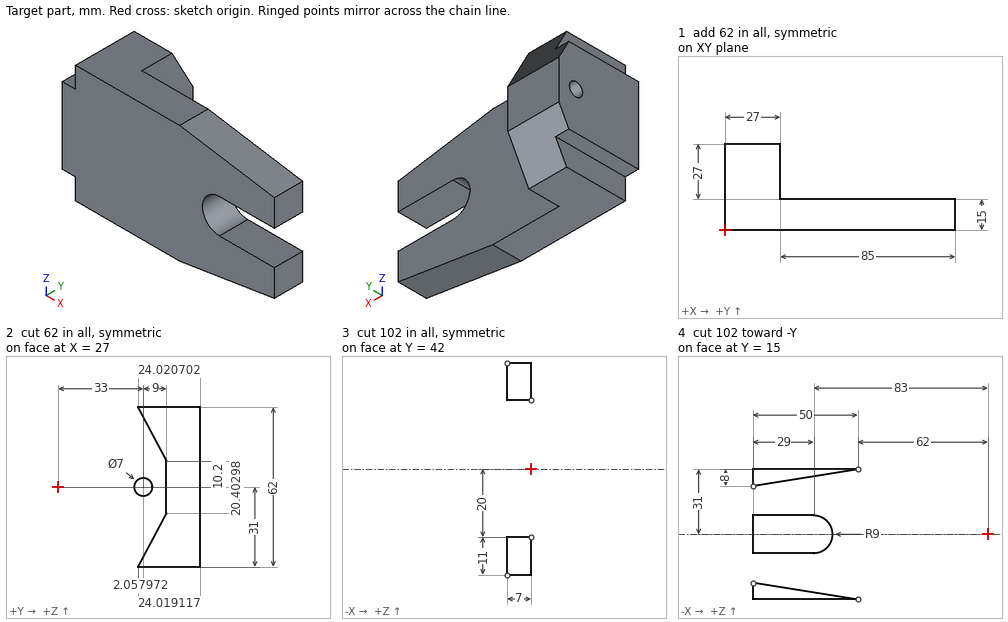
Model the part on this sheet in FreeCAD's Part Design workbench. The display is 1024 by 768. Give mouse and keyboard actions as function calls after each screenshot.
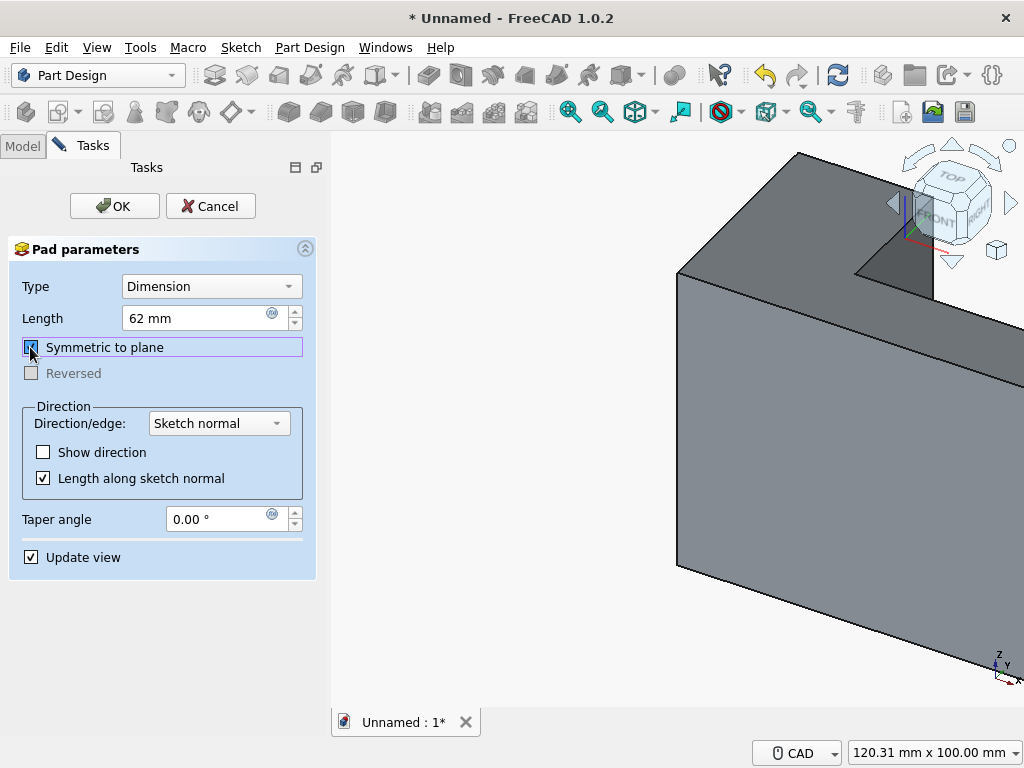
click(115, 206)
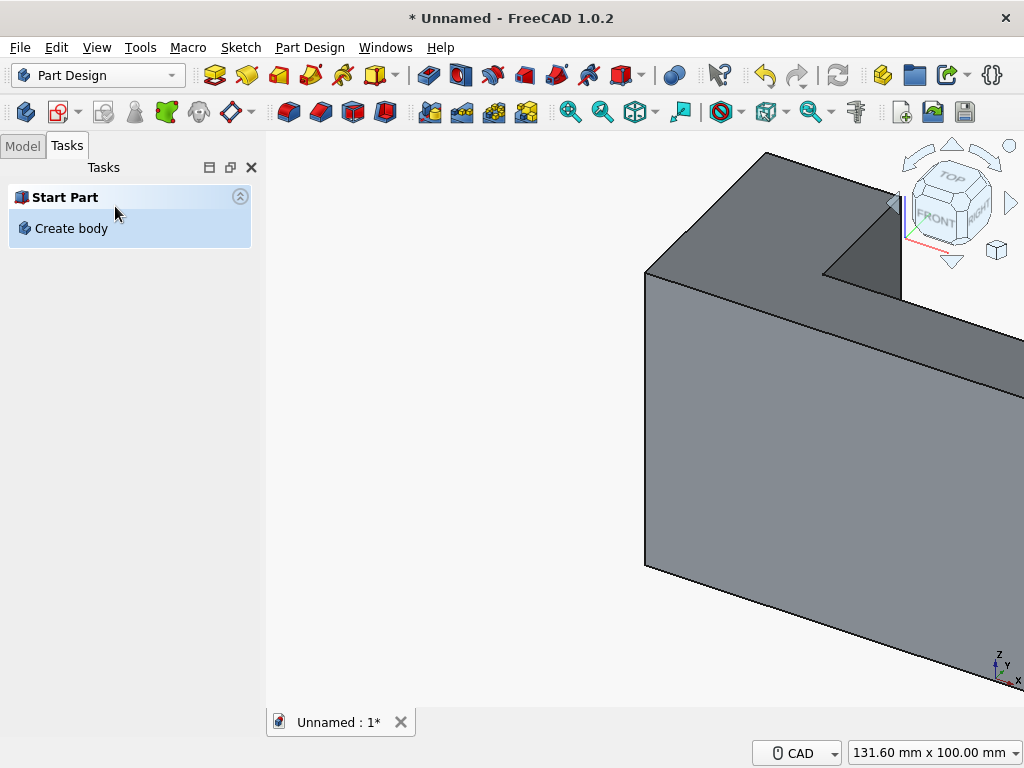
click(572, 112)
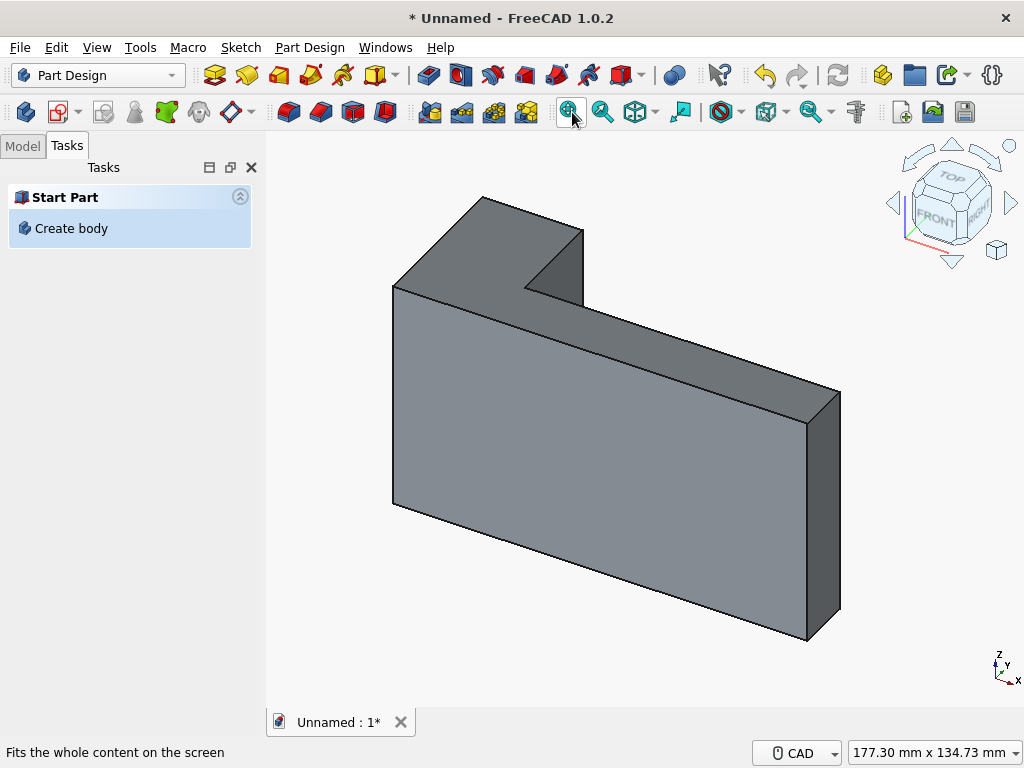
key(0)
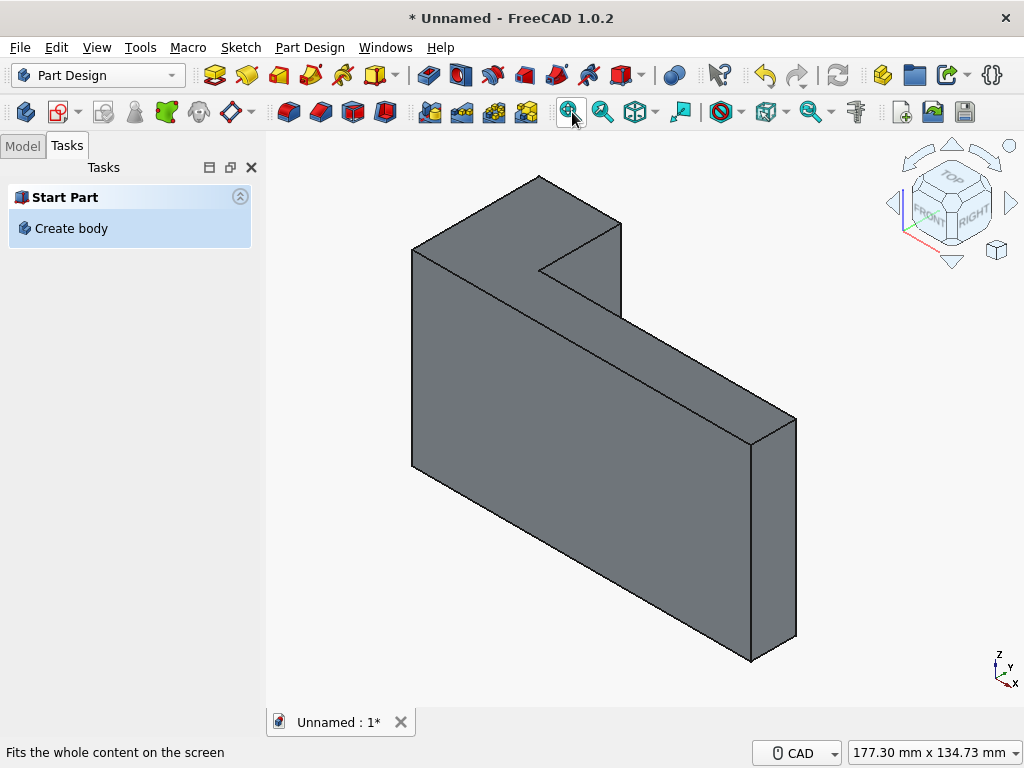
key(3)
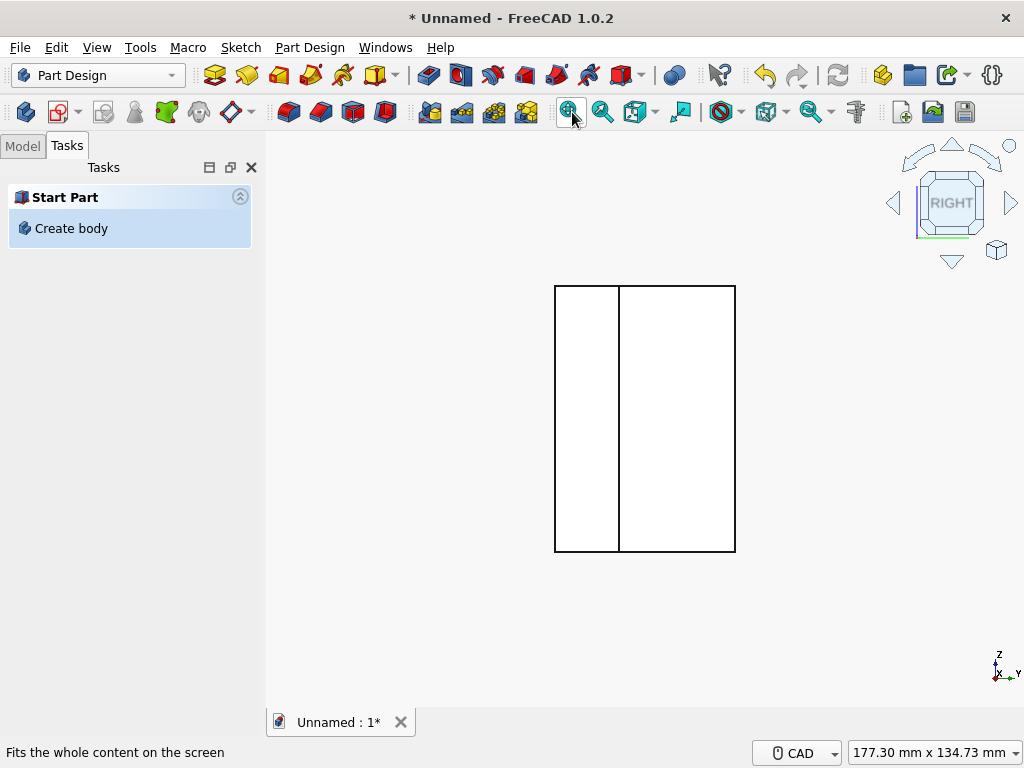
click(677, 380)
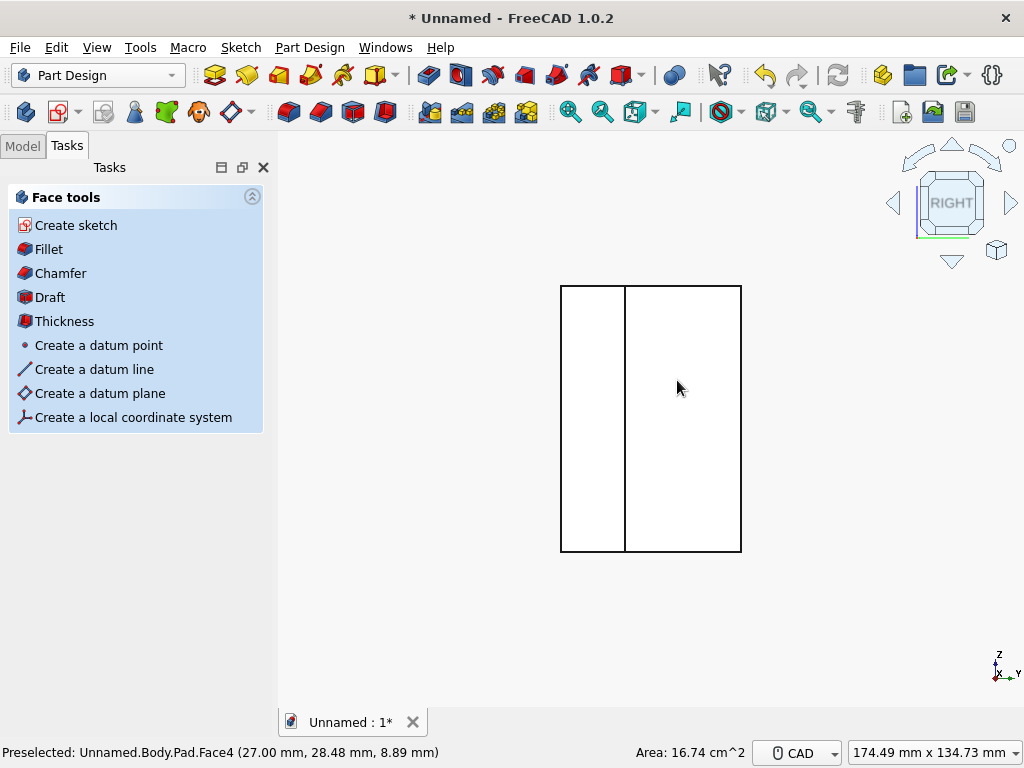
click(58, 112)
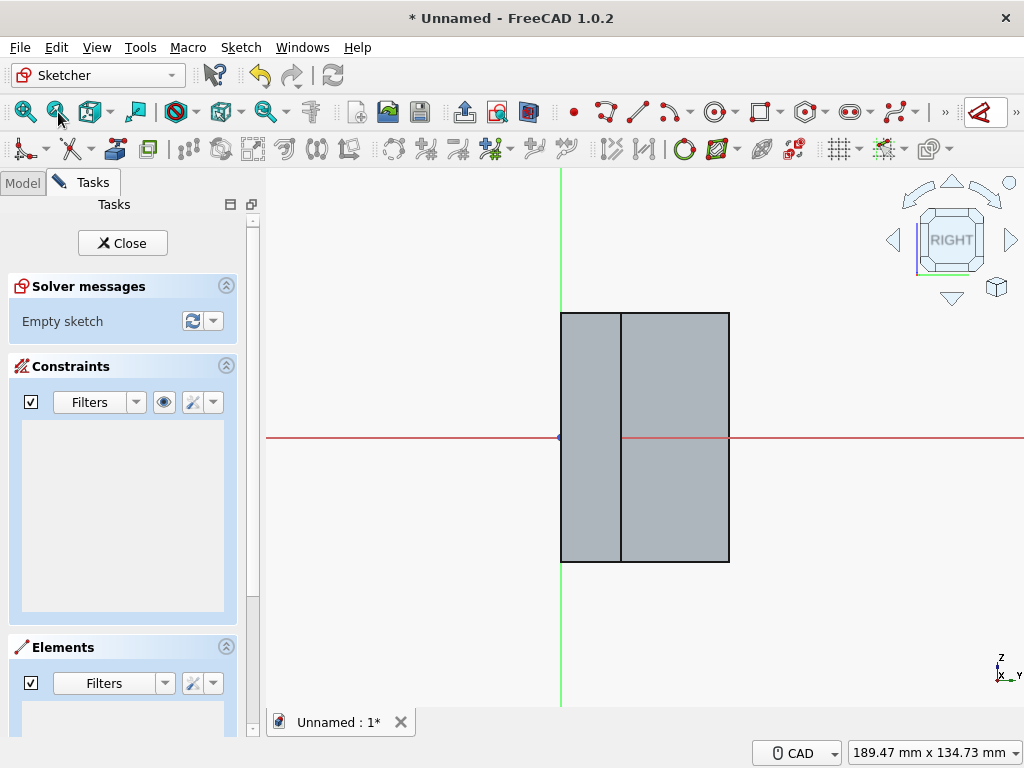
scroll(859, 438, up, 2)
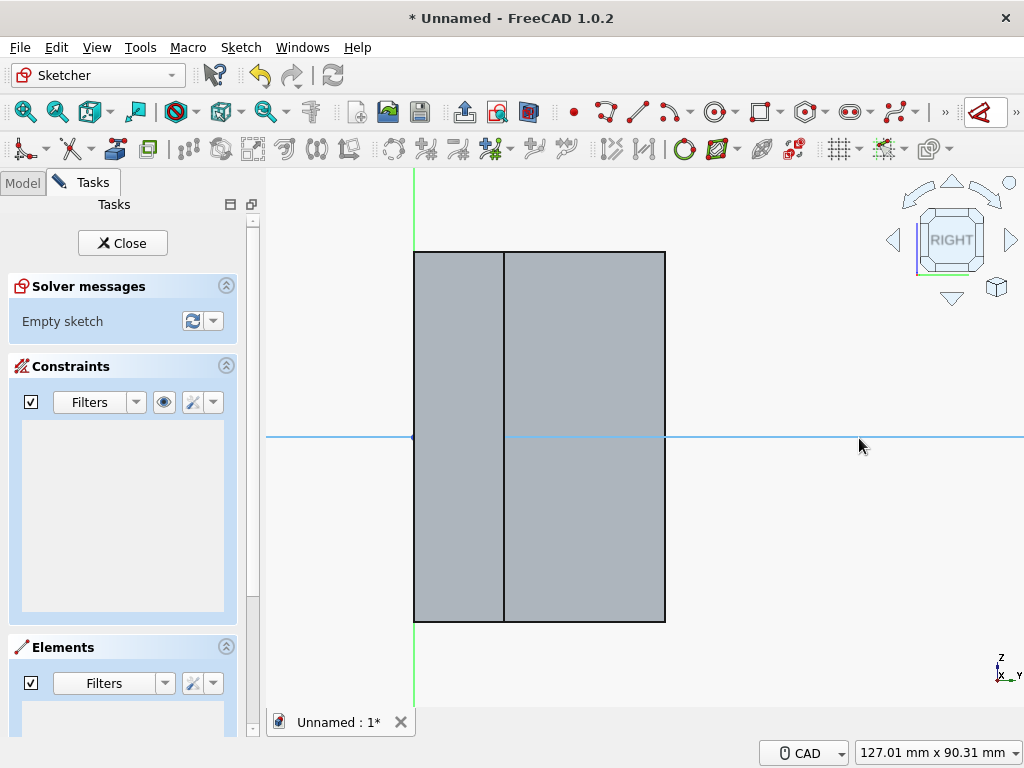
click(606, 112)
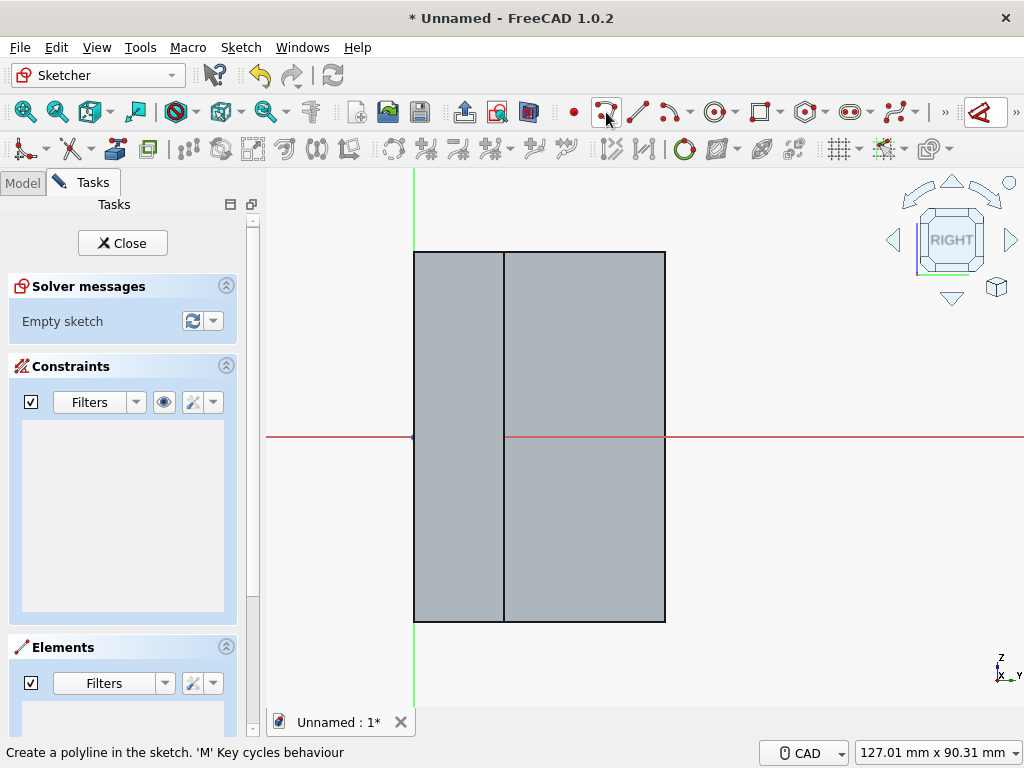
click(665, 376)
click(665, 498)
click(599, 622)
click(742, 622)
click(742, 252)
click(599, 252)
click(665, 377)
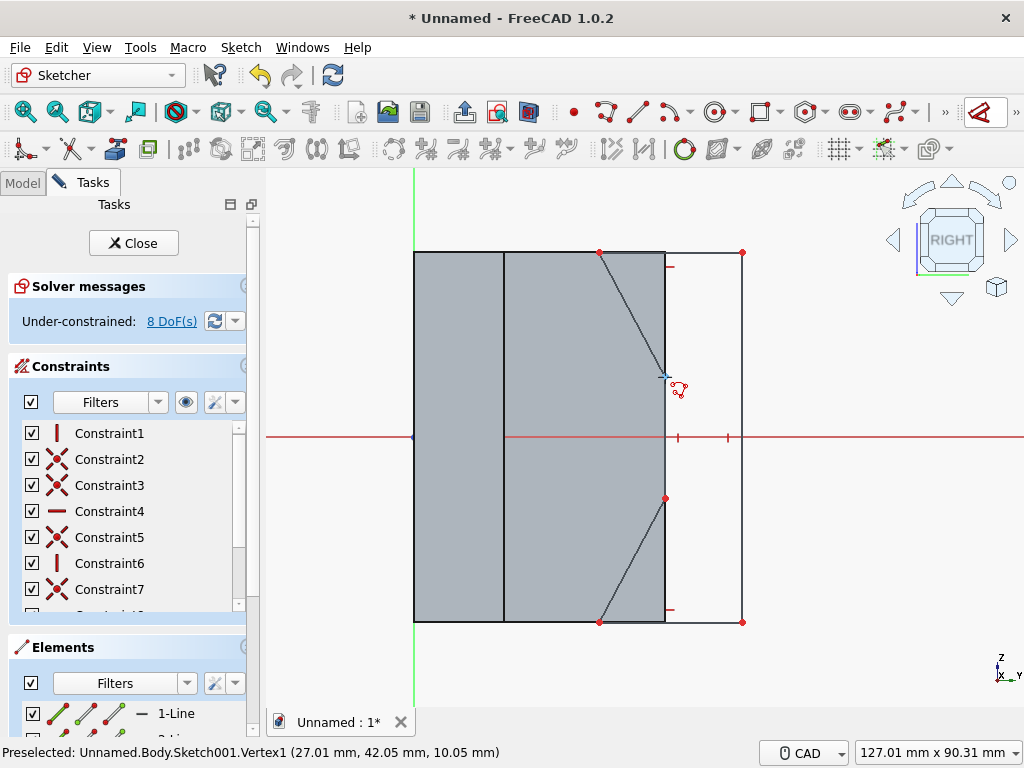
click(716, 112)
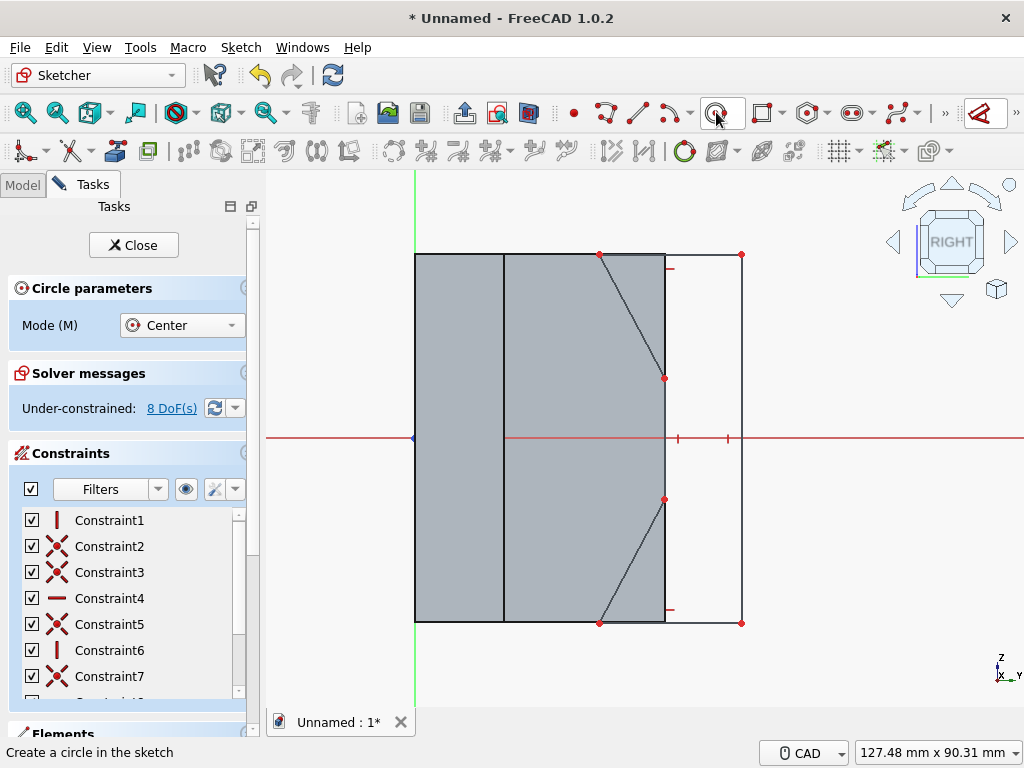
click(611, 438)
click(626, 423)
key(Escape)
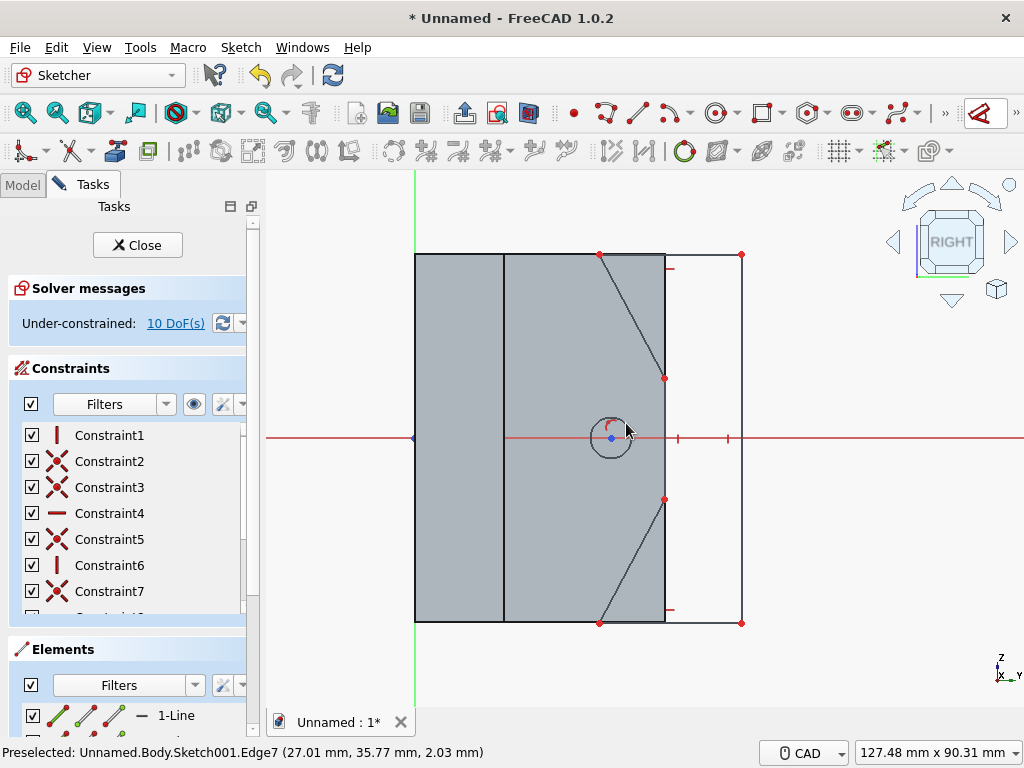
click(625, 423)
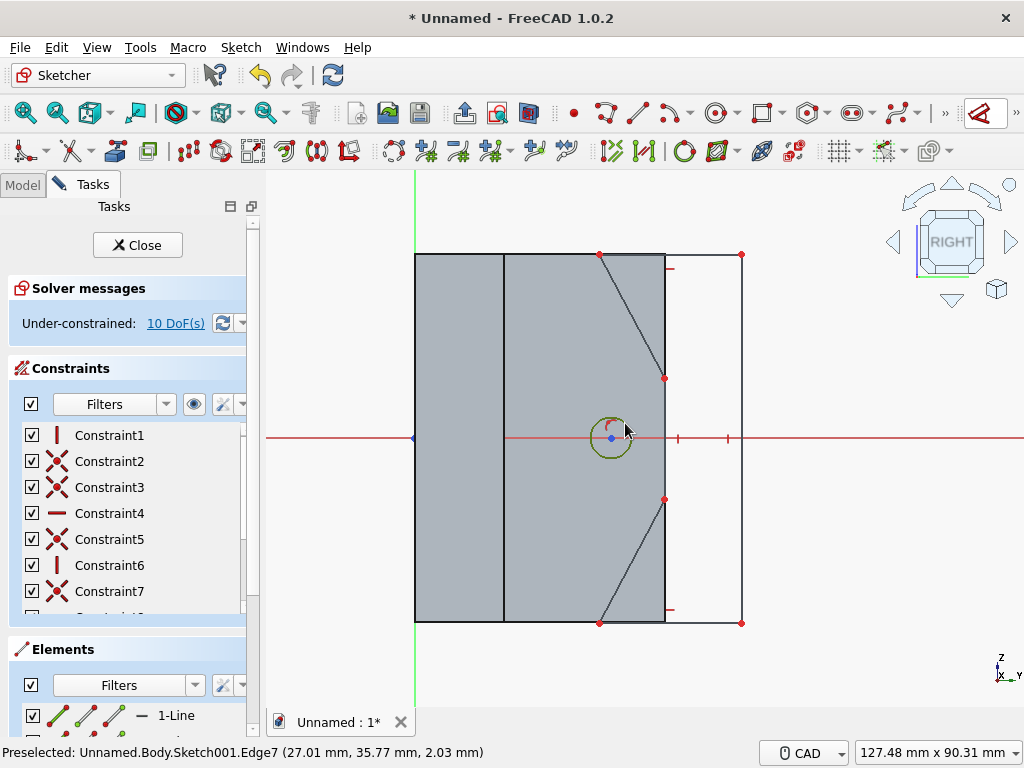
click(1002, 114)